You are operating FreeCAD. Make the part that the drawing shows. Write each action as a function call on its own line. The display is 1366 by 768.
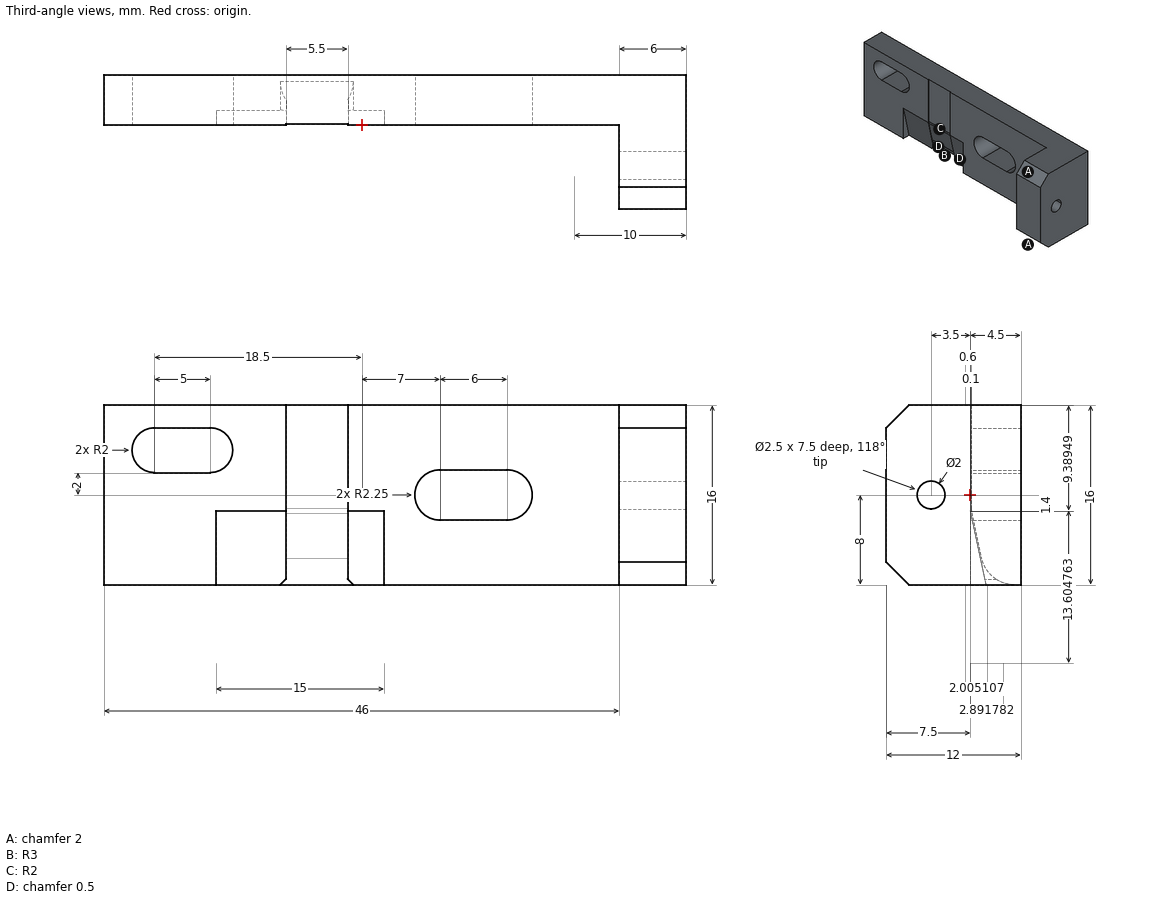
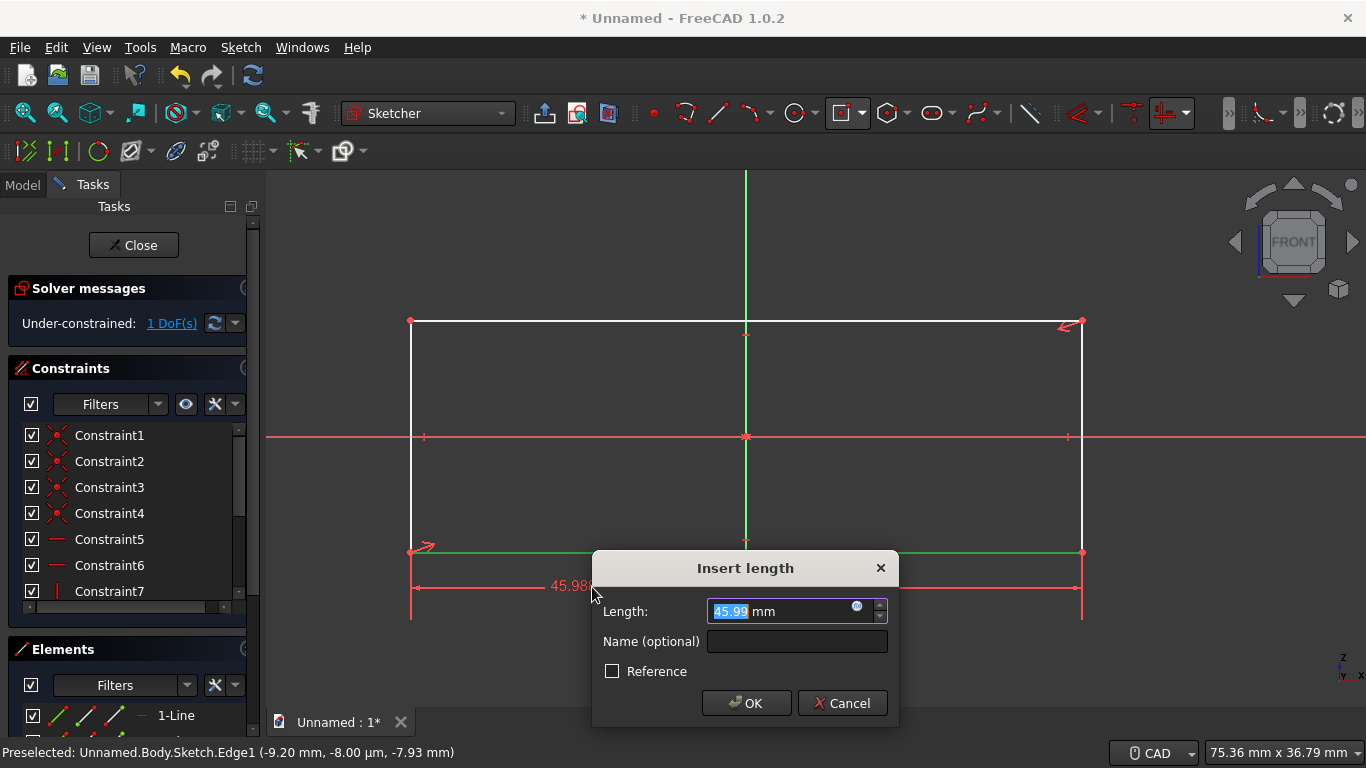
text(46)
key(Return)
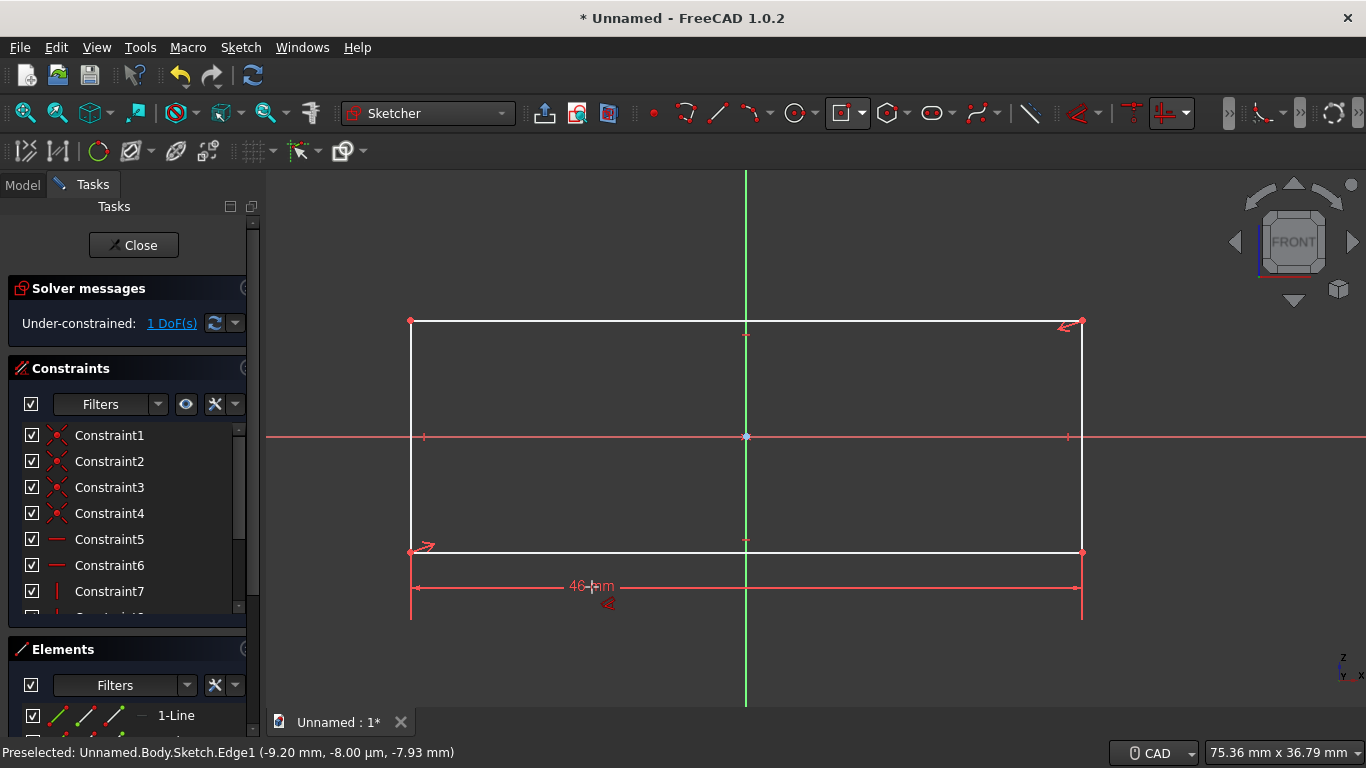
click(1082, 483)
click(1116, 384)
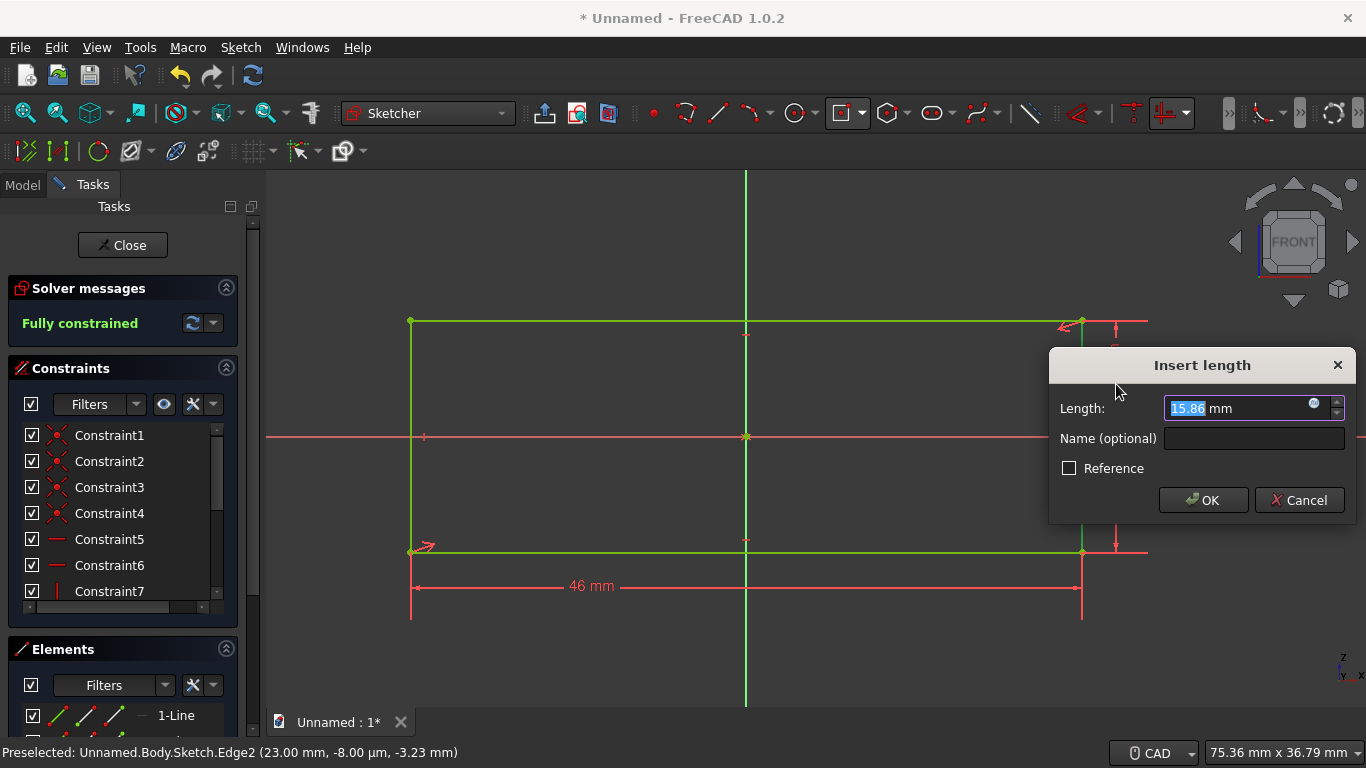
text(16)
key(Return)
key(Escape)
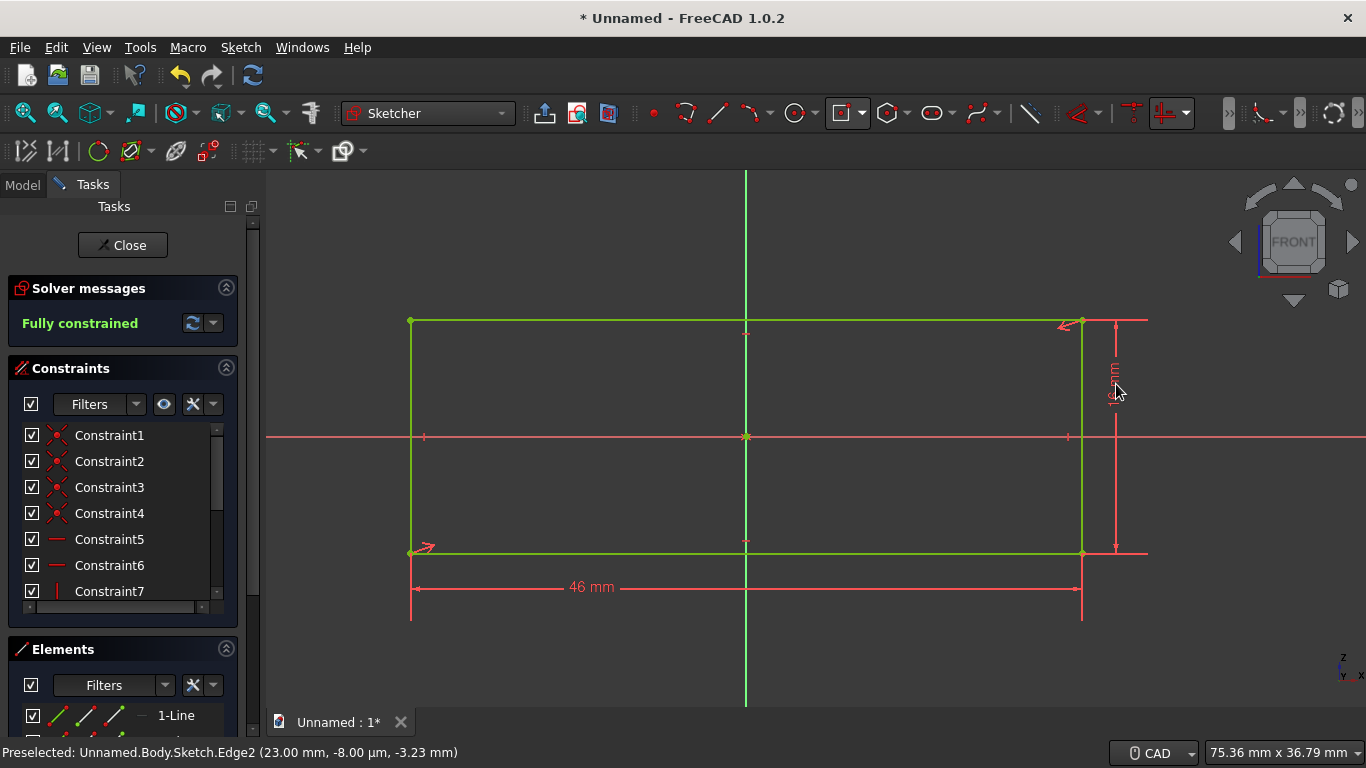
click(123, 245)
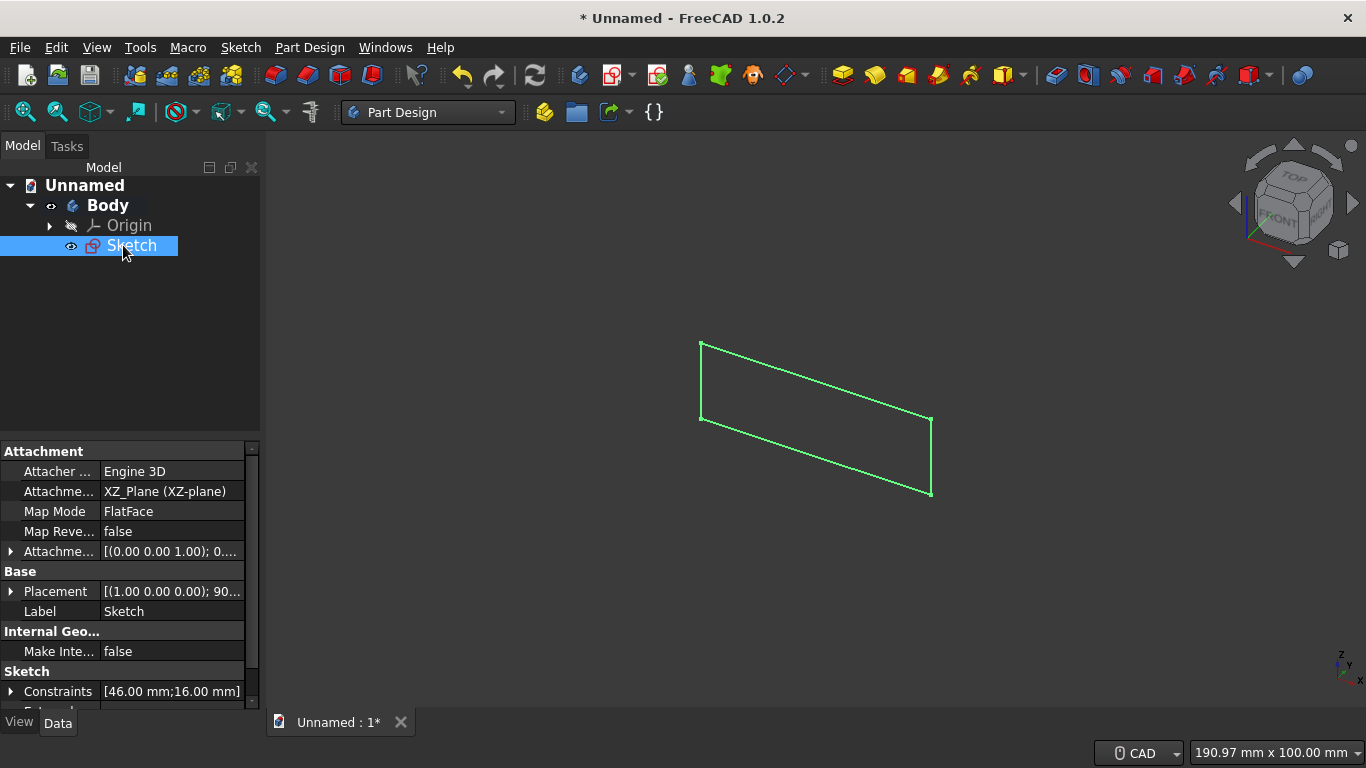
click(844, 76)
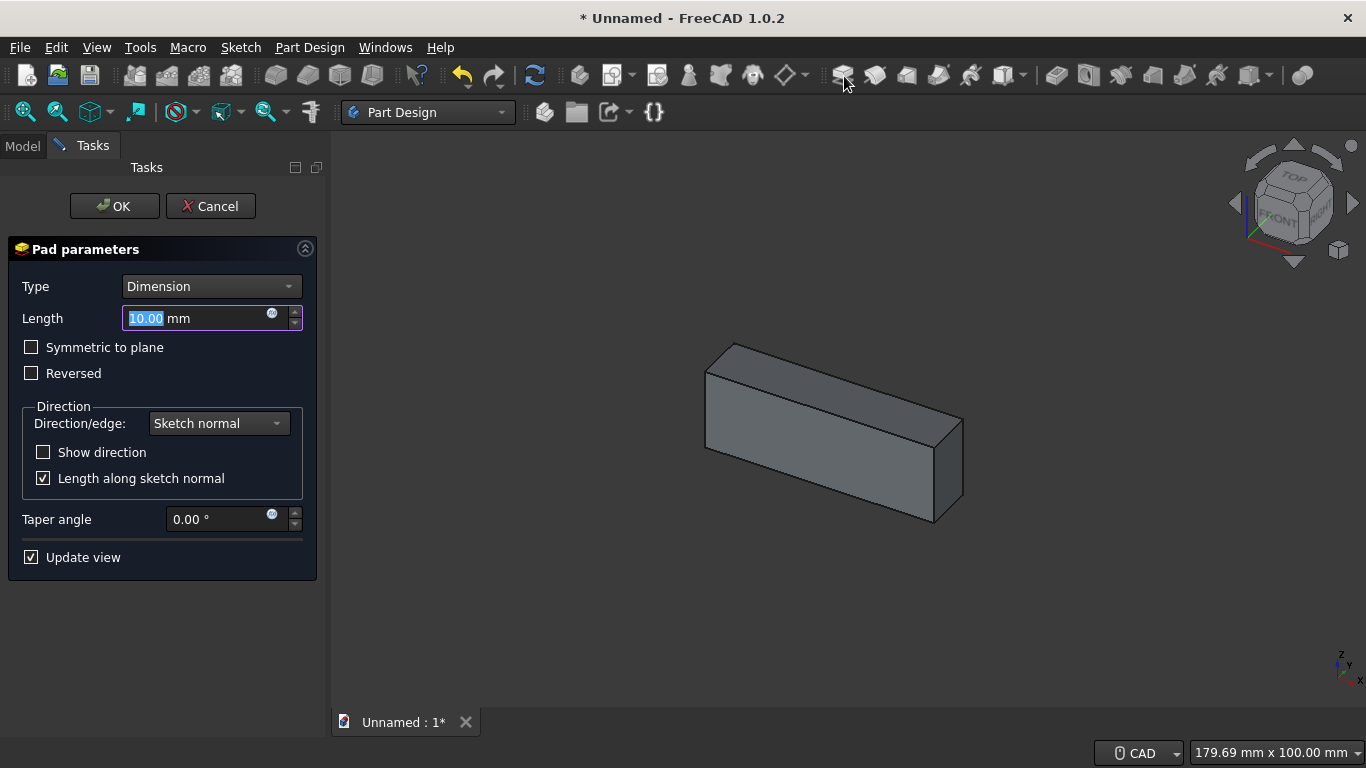
text(4.5)
key(Tab)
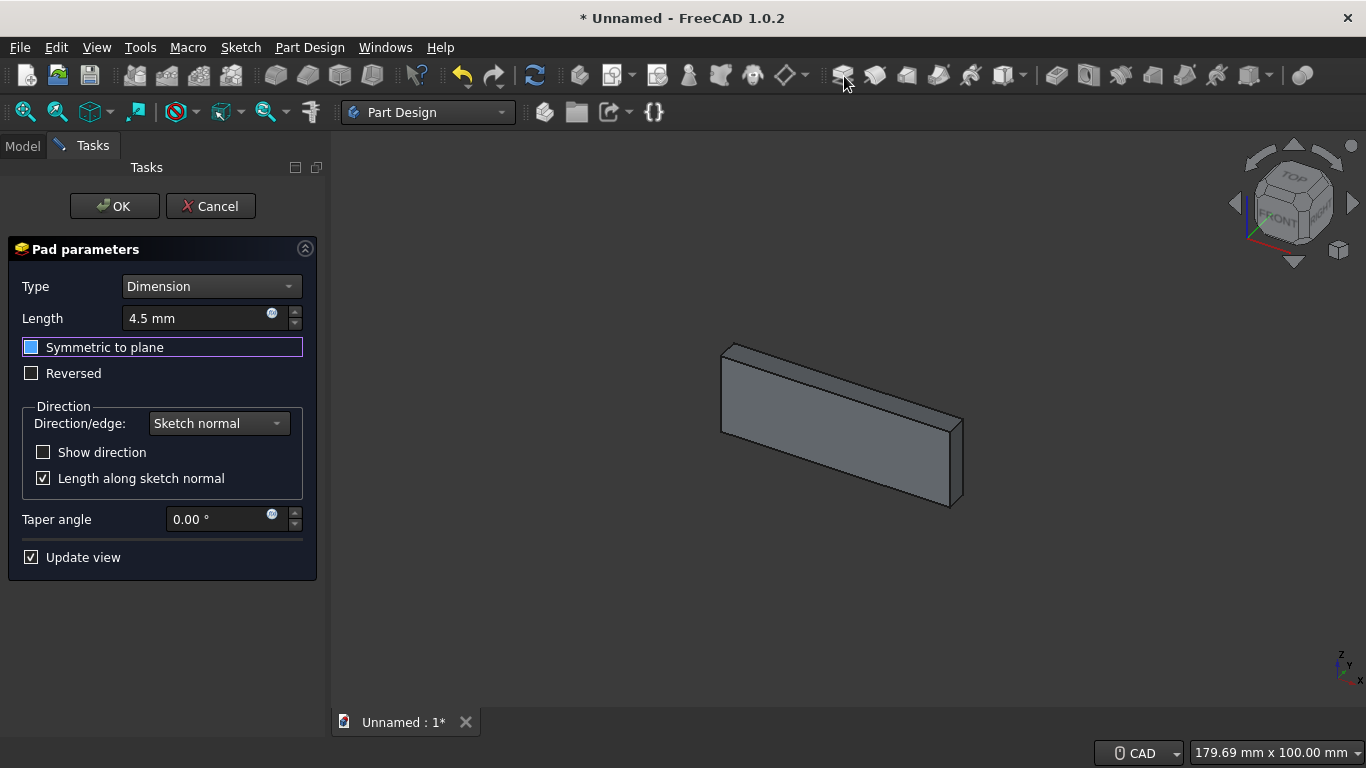
click(30, 373)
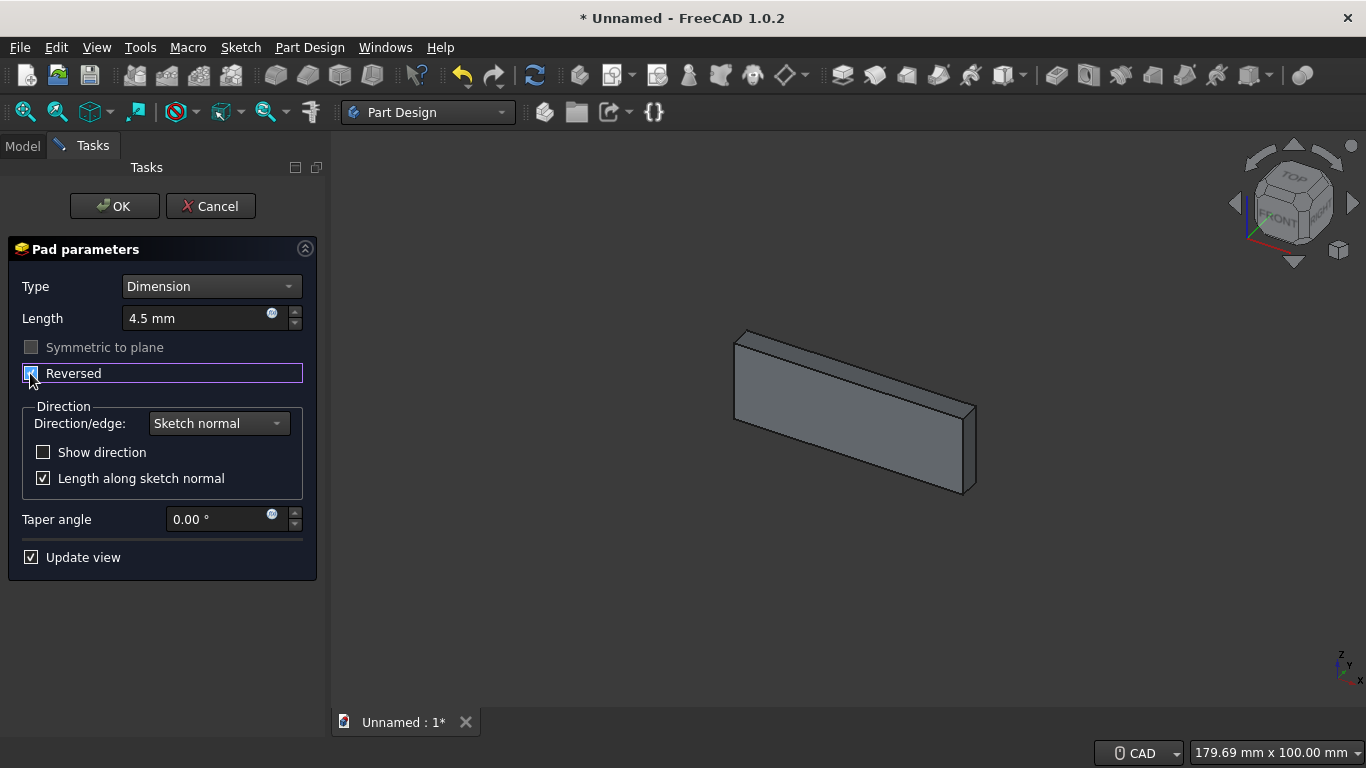
click(115, 206)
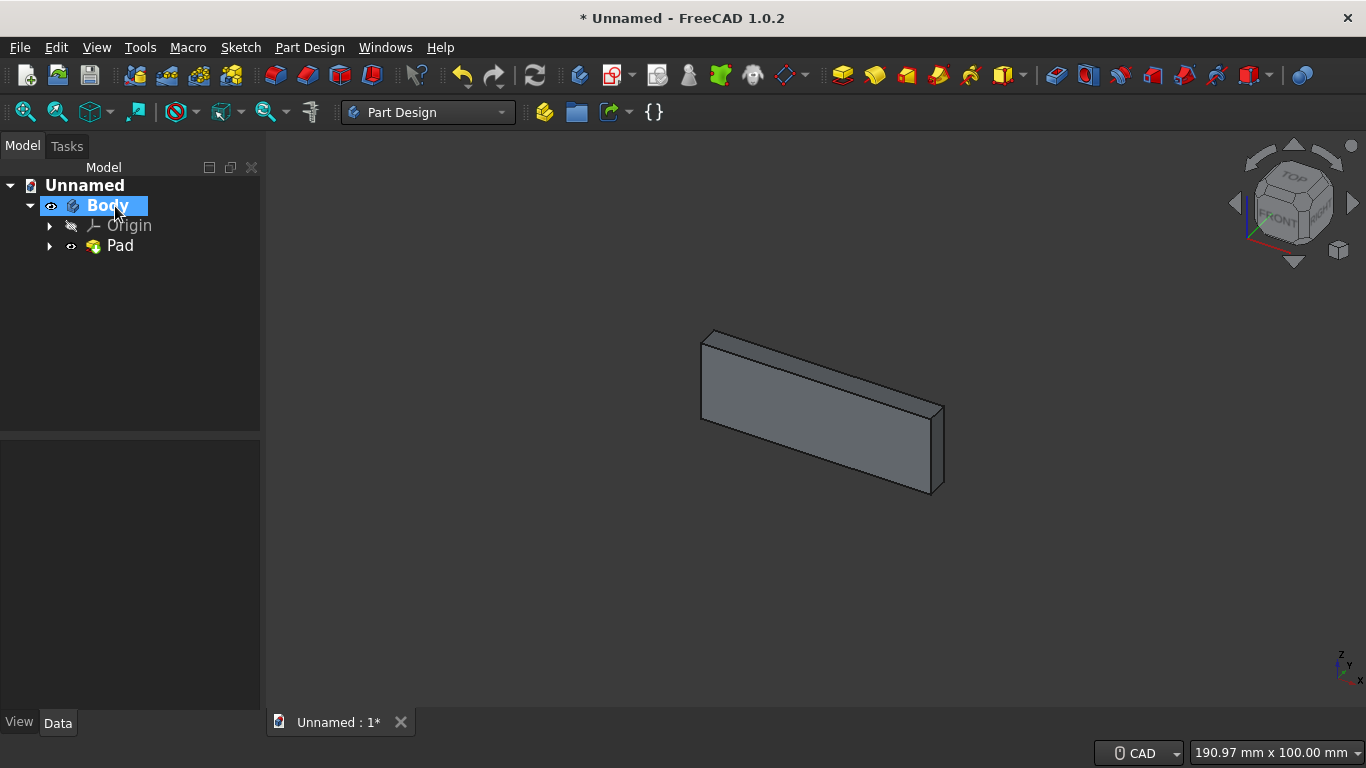
click(26, 112)